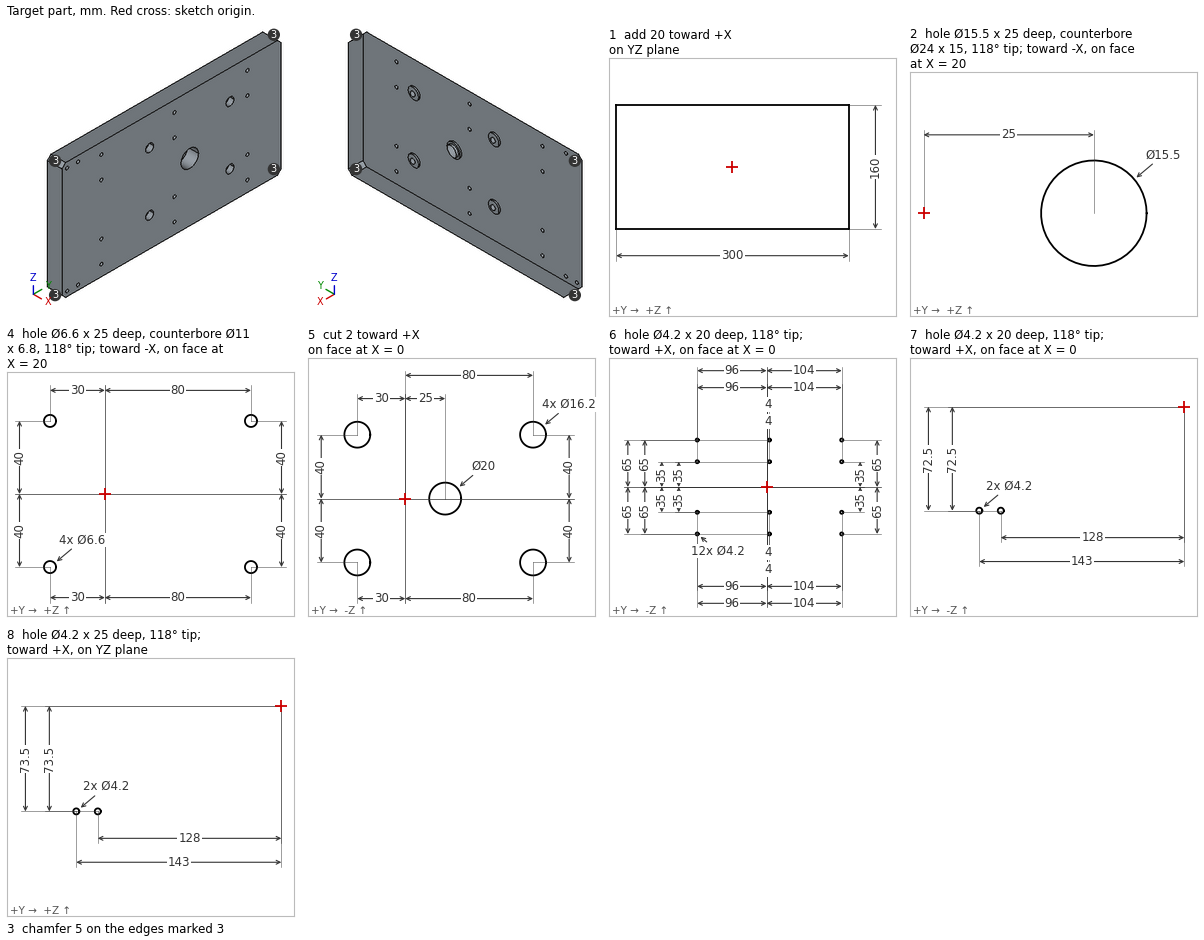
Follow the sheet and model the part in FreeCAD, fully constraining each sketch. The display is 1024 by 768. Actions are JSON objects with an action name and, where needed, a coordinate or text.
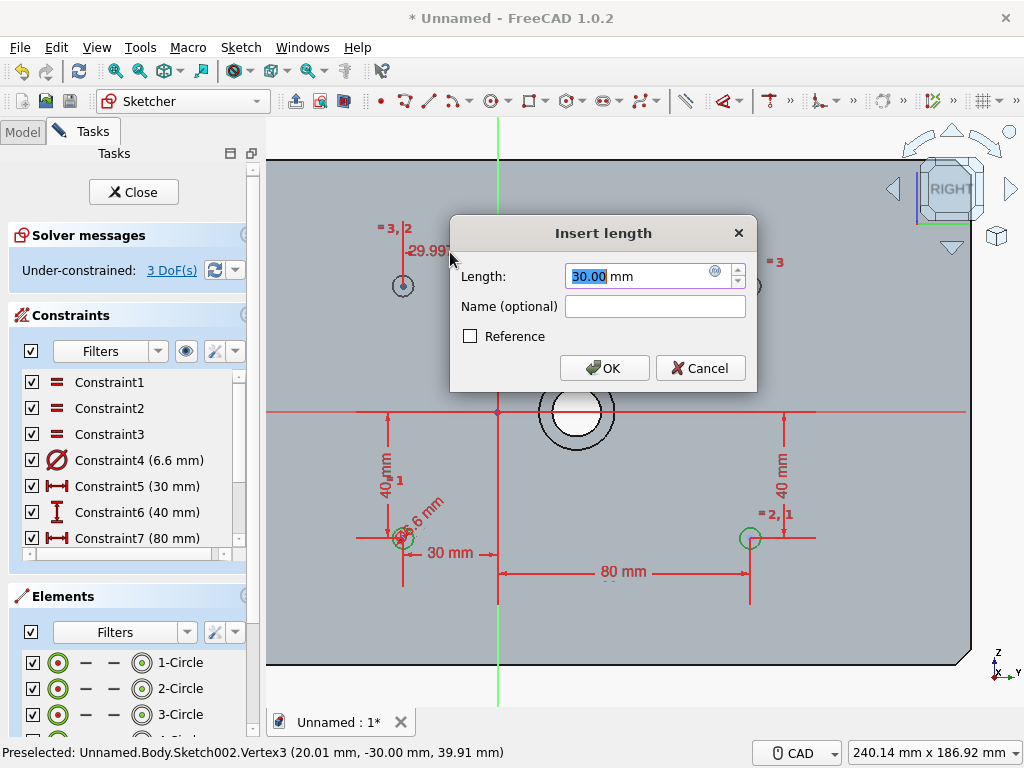
{"action": "type", "text": "30"}
{"action": "key", "text": "Return"}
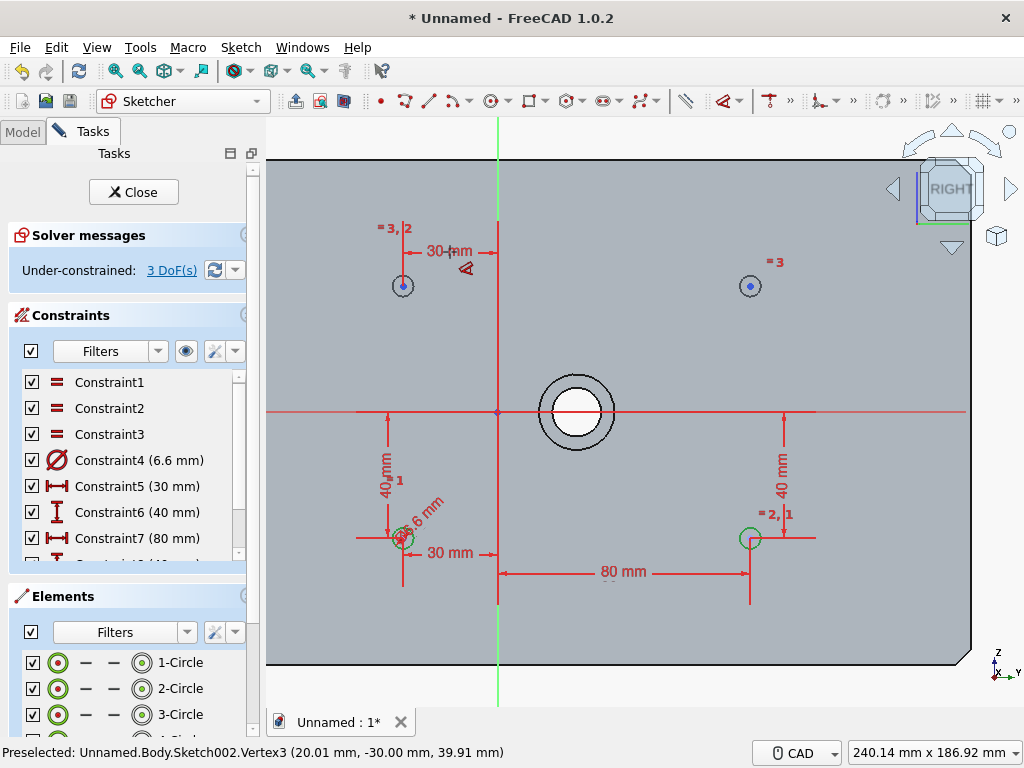
{"action": "left_click", "coordinate": [403, 286]}
{"action": "left_click", "coordinate": [369, 349]}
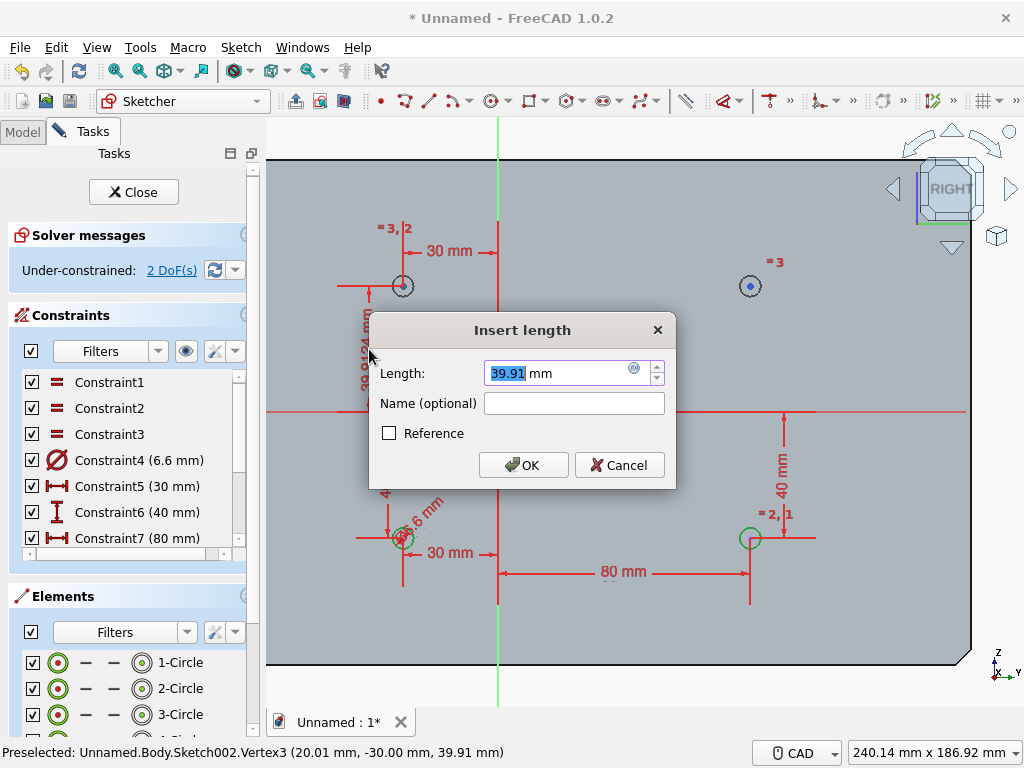
{"action": "type", "text": "40"}
{"action": "key", "text": "Return"}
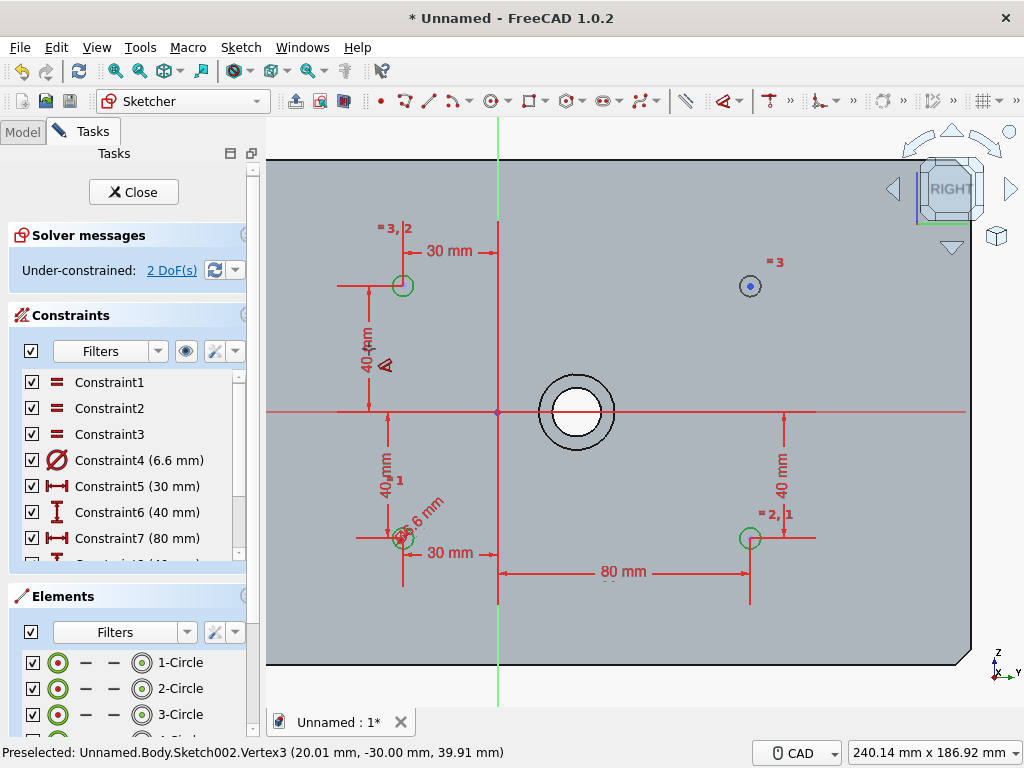
{"action": "left_click", "coordinate": [750, 286]}
{"action": "left_click", "coordinate": [624, 252]}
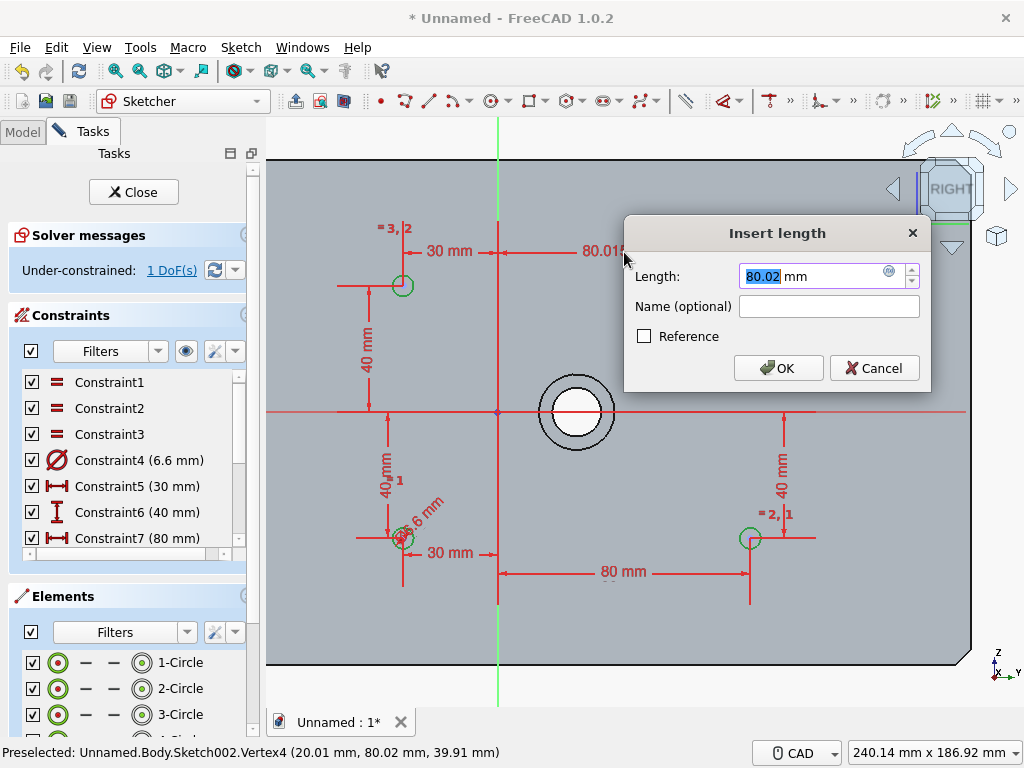
{"action": "type", "text": "80"}
{"action": "key", "text": "Return"}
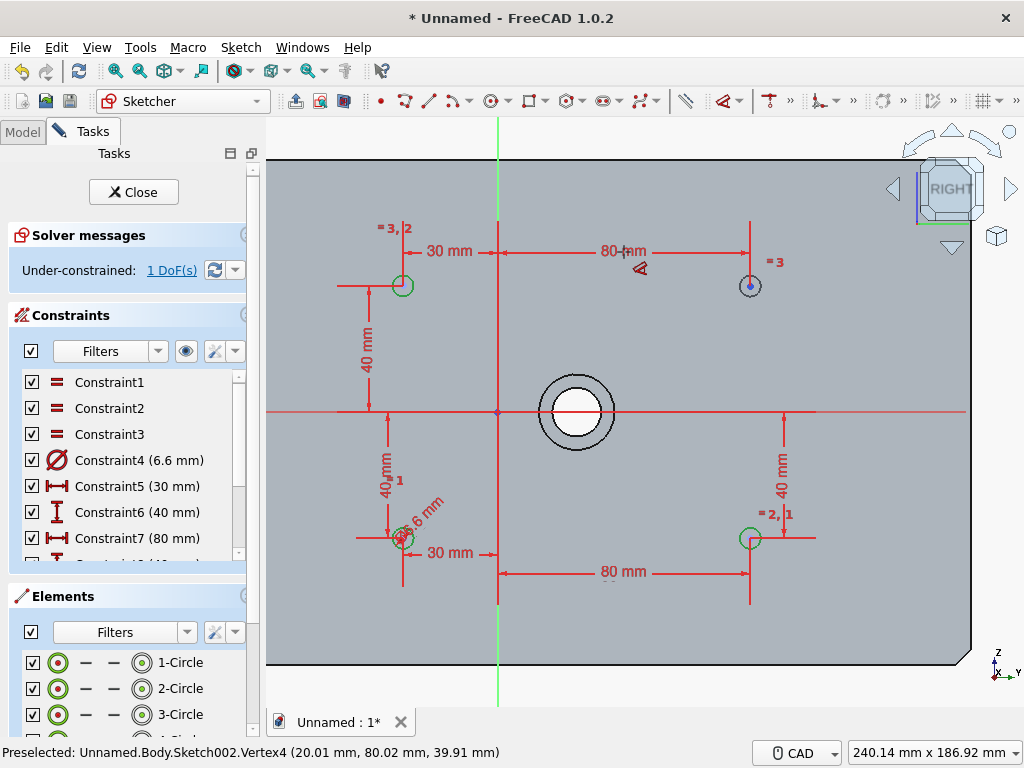
{"action": "left_click", "coordinate": [750, 286]}
{"action": "left_click", "coordinate": [784, 349]}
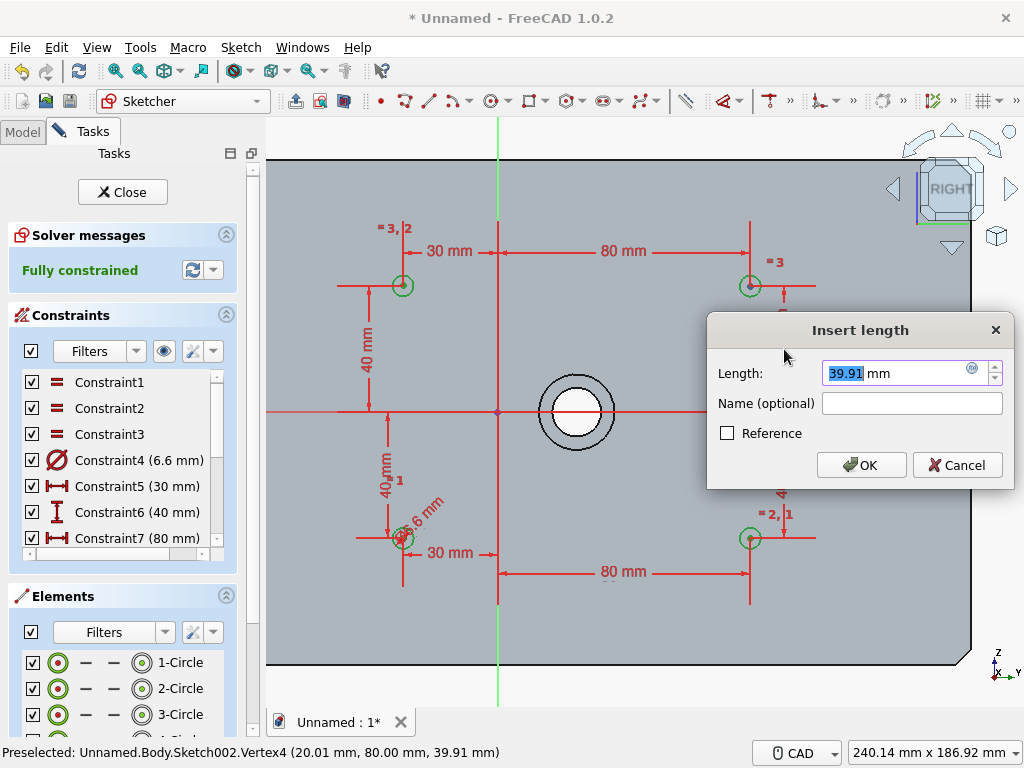
{"action": "type", "text": "40"}
{"action": "key", "text": "Return"}
{"action": "key", "text": "Escape"}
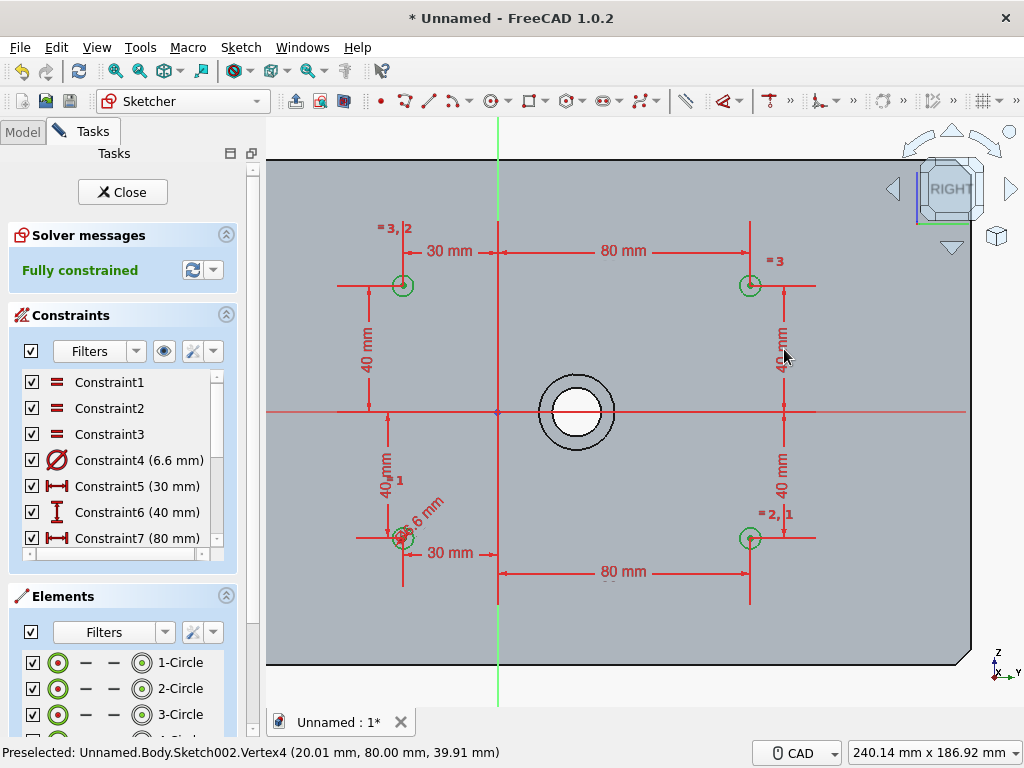
{"action": "left_click", "coordinate": [123, 192]}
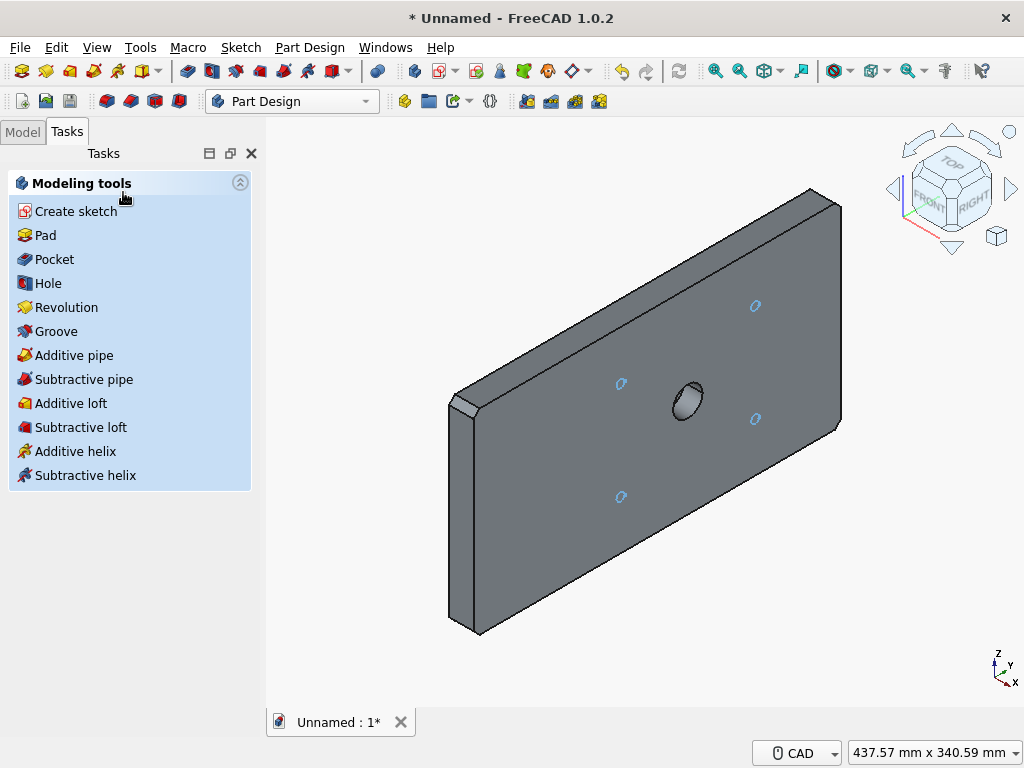
{"action": "left_click", "coordinate": [212, 72]}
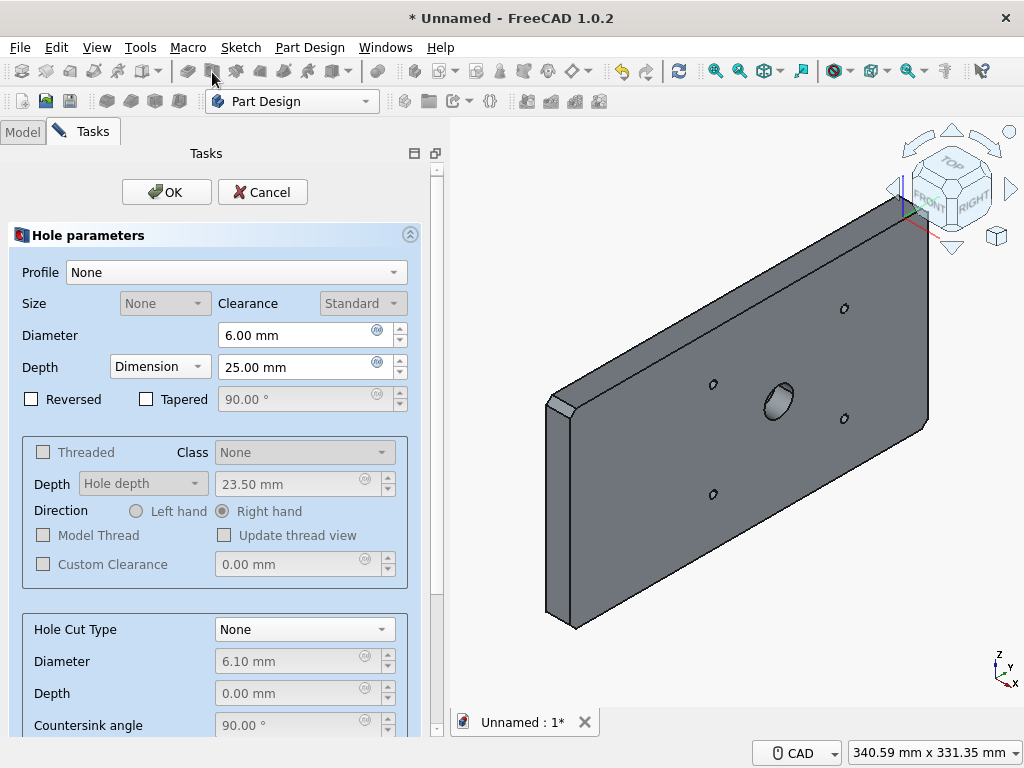
{"action": "triple_click", "coordinate": [305, 335]}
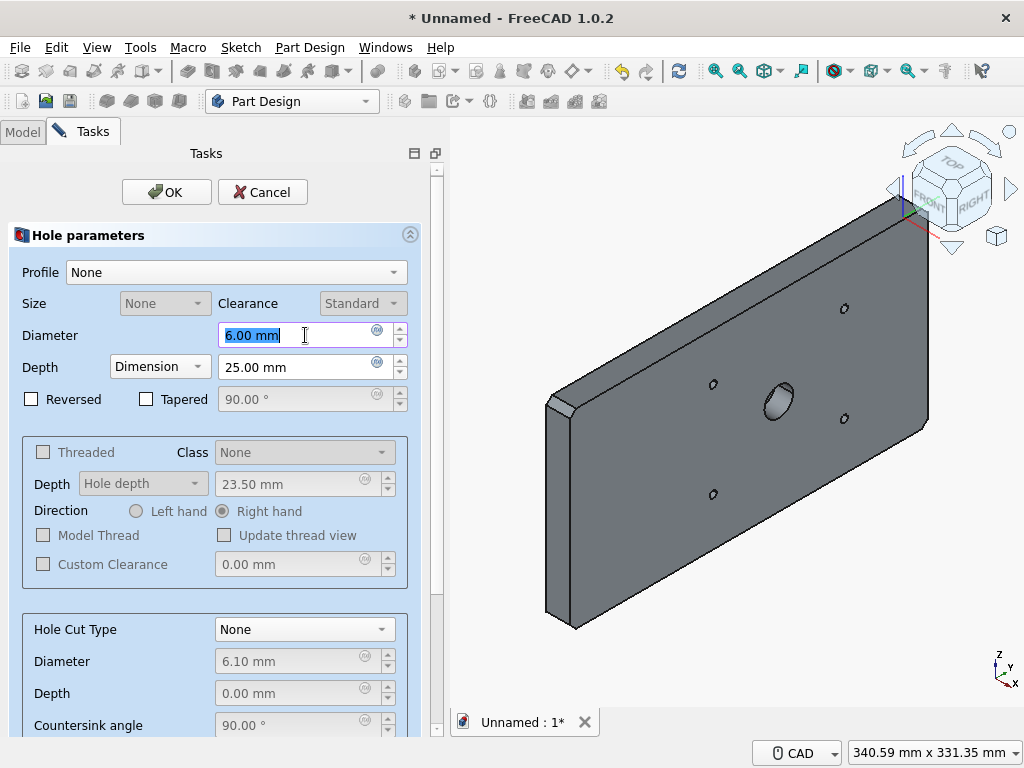
{"action": "type", "text": "6.6"}
{"action": "key", "text": "Tab"}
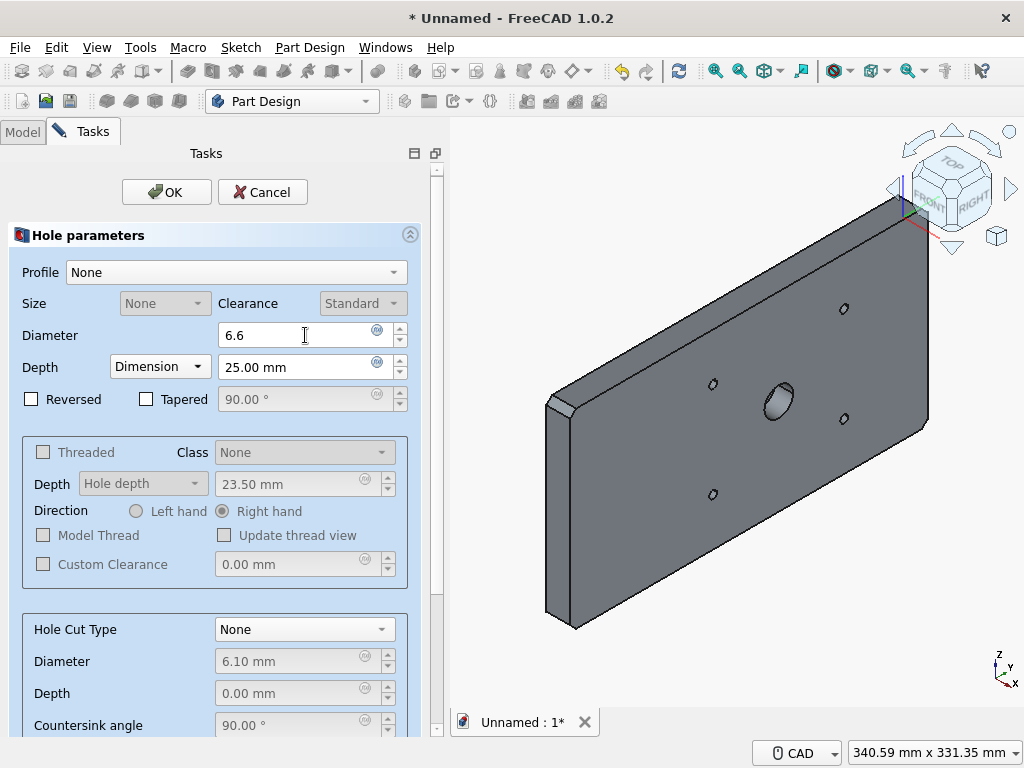
{"action": "triple_click", "coordinate": [305, 367]}